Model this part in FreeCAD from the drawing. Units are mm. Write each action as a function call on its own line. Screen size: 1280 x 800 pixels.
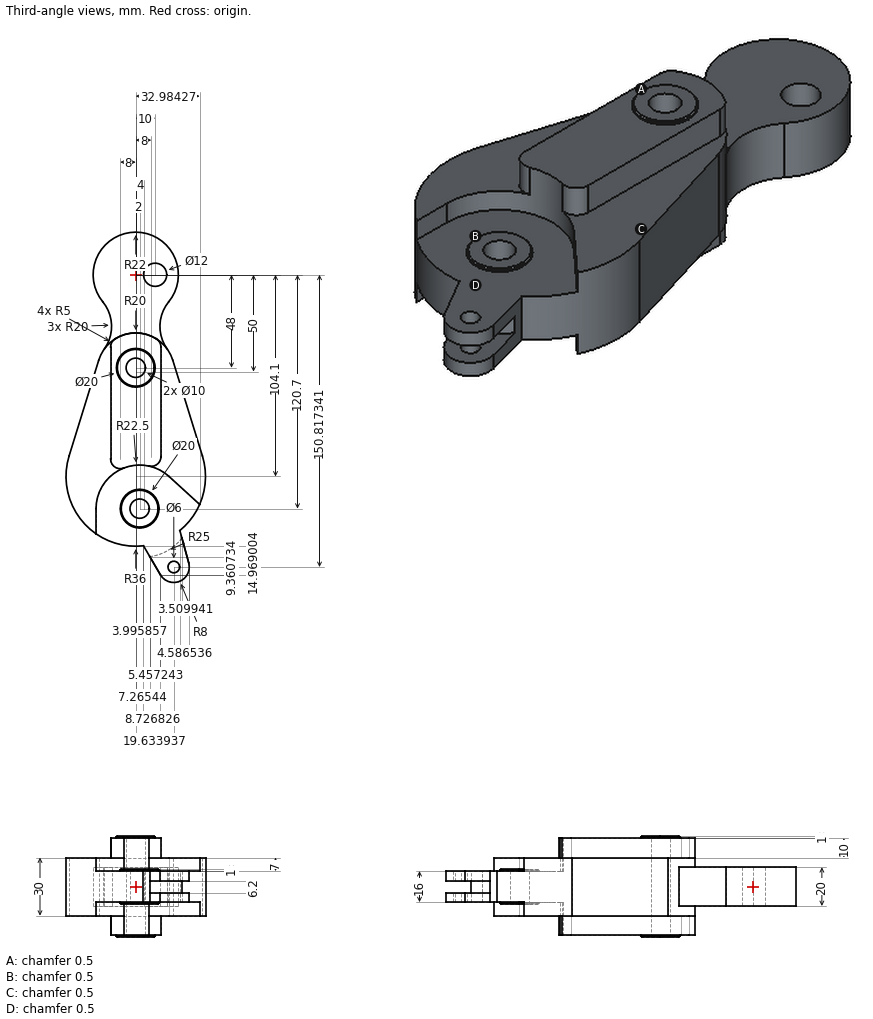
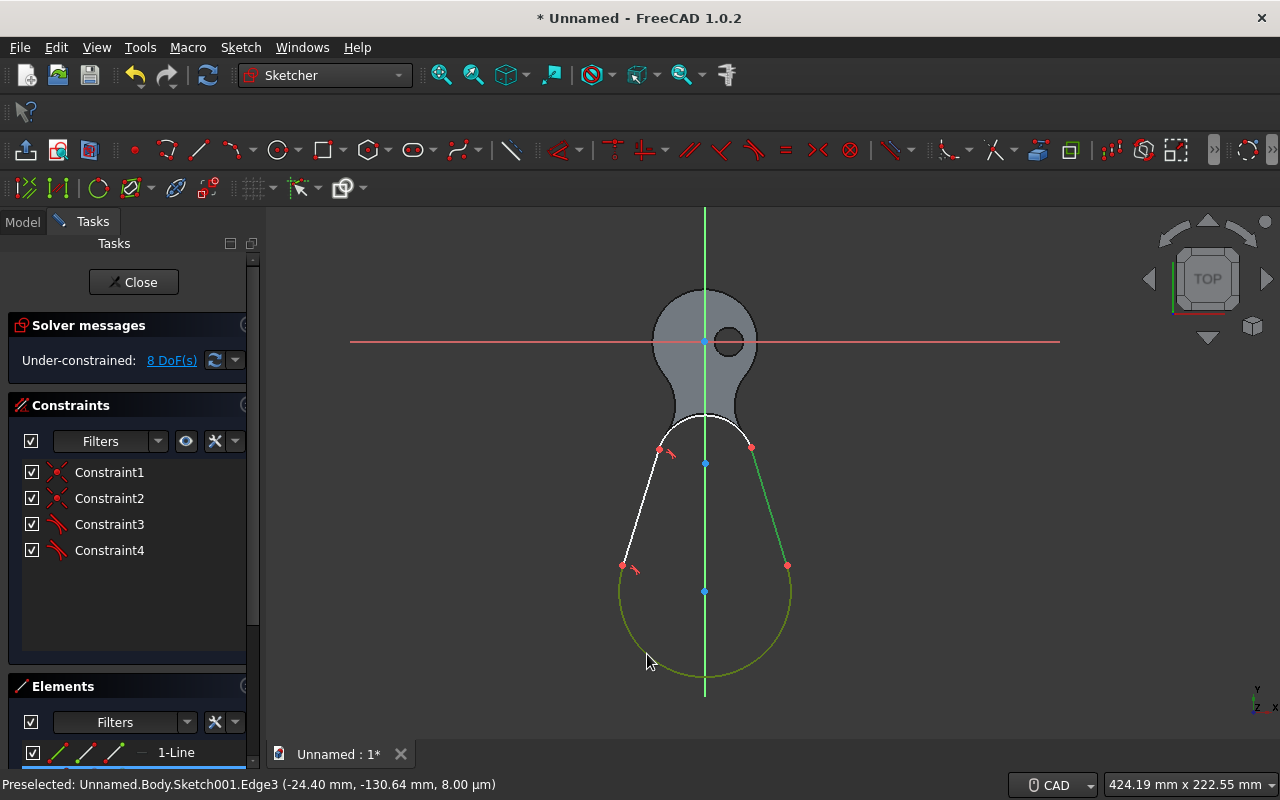
click(754, 150)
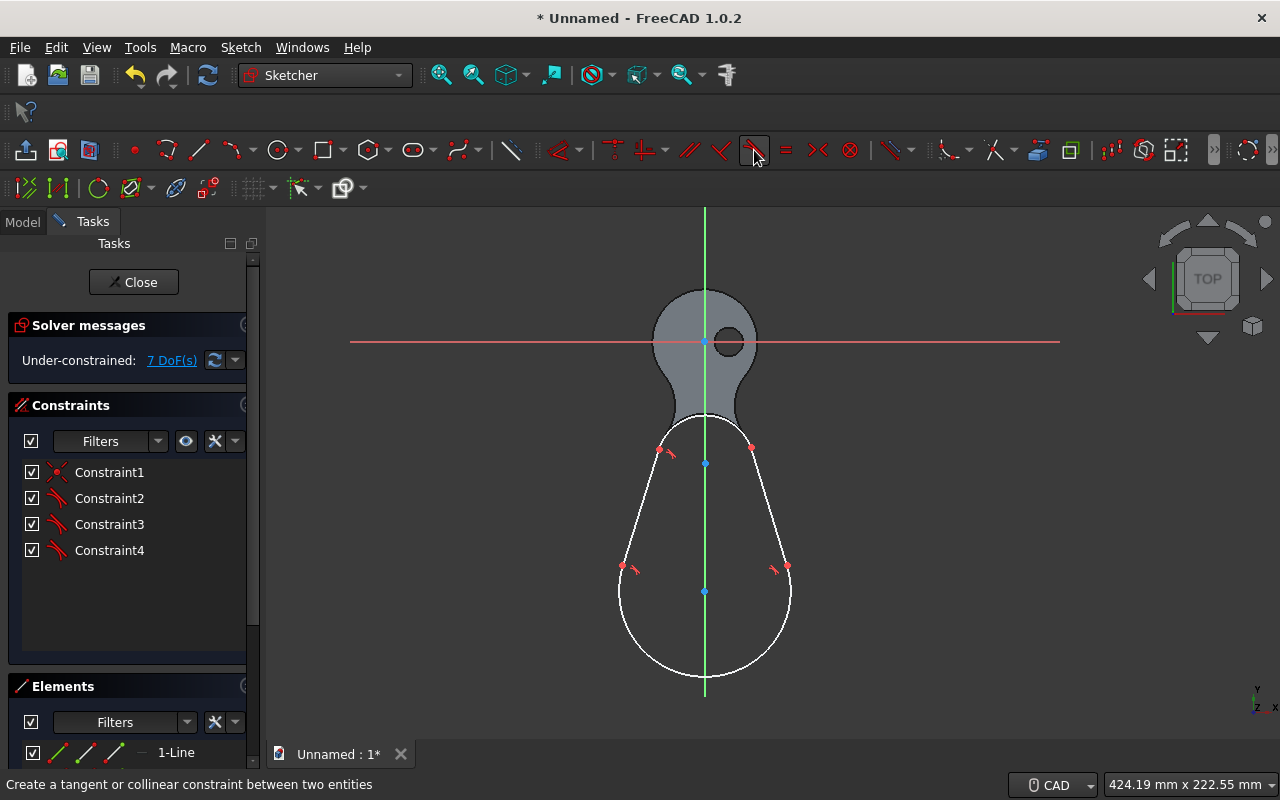
click(776, 531)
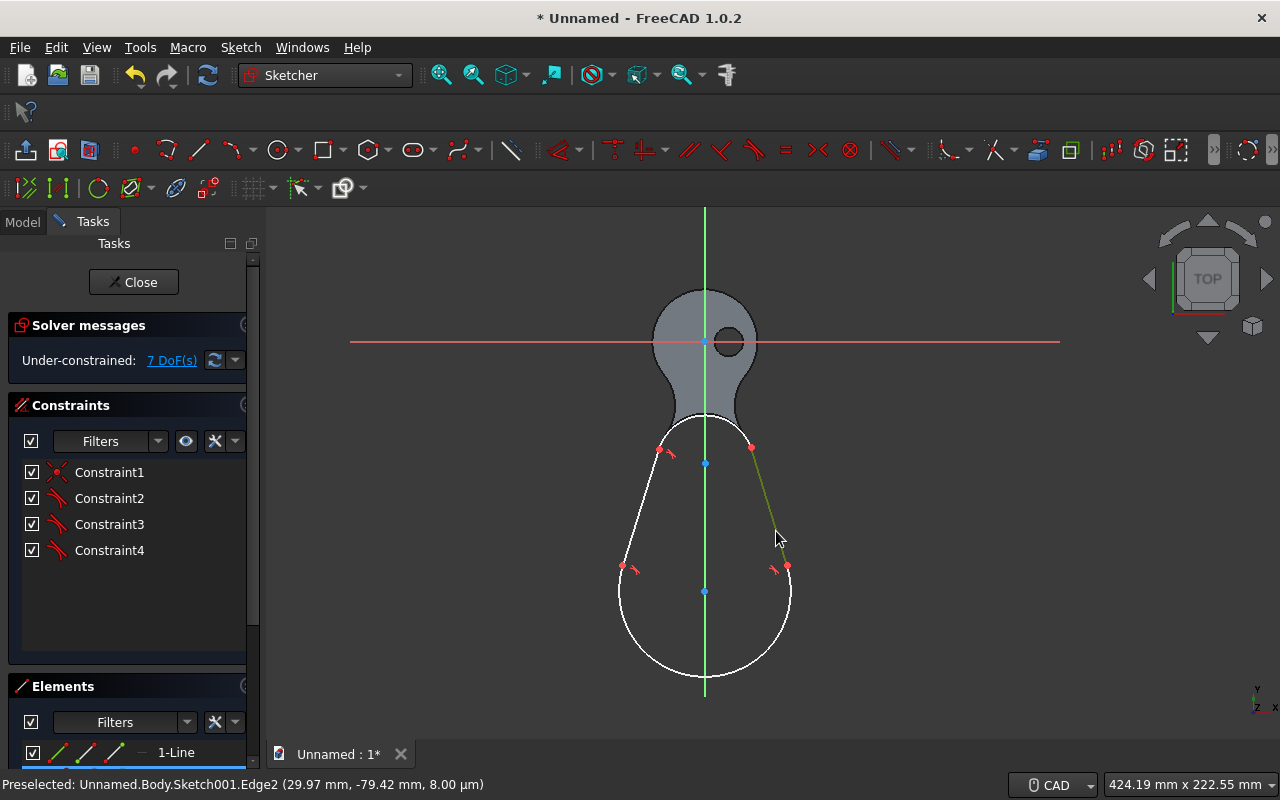
click(728, 421)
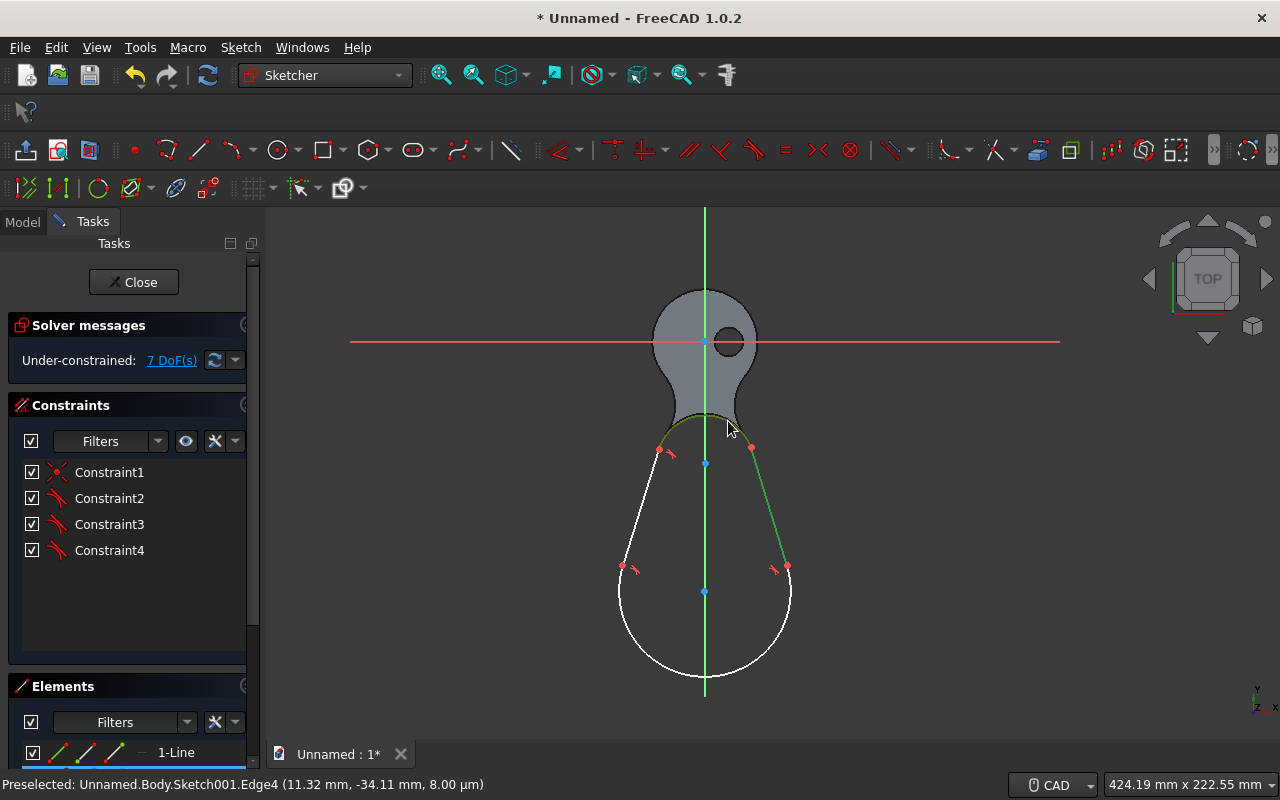
click(754, 150)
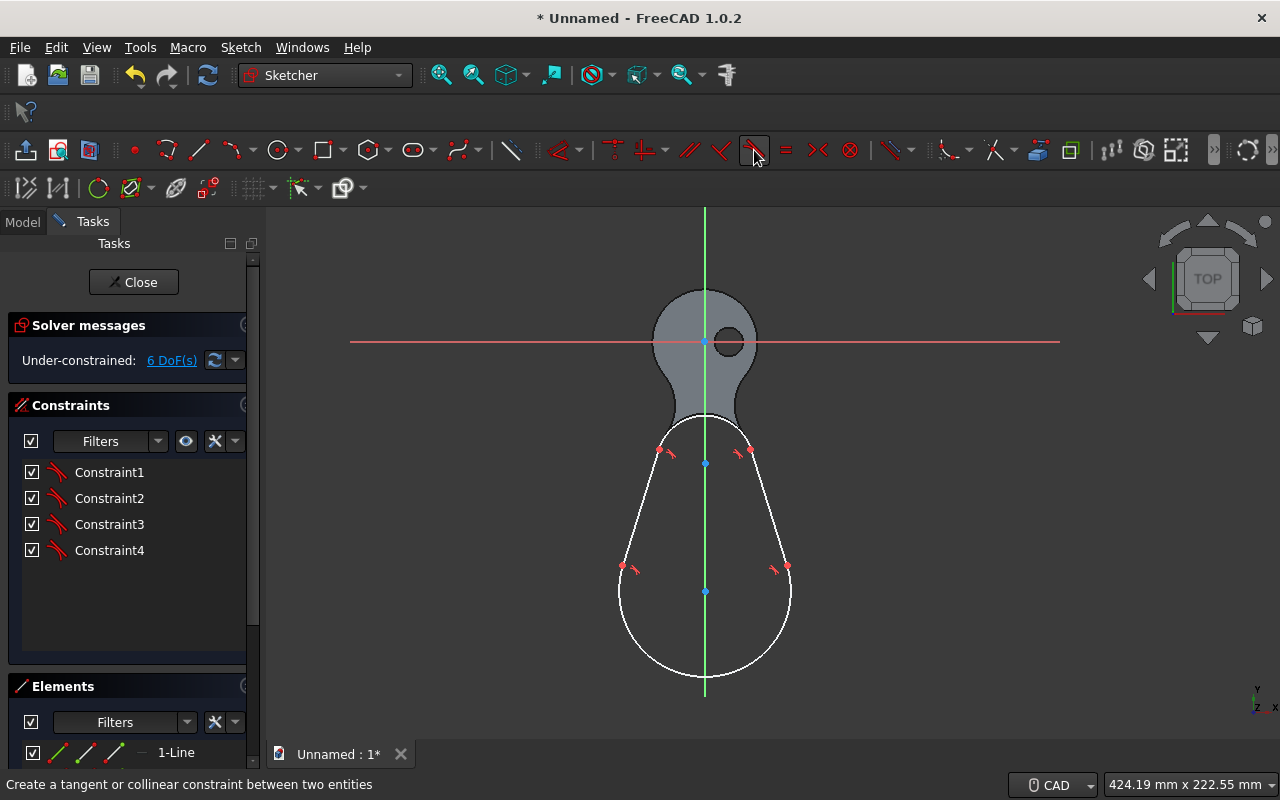
click(705, 591)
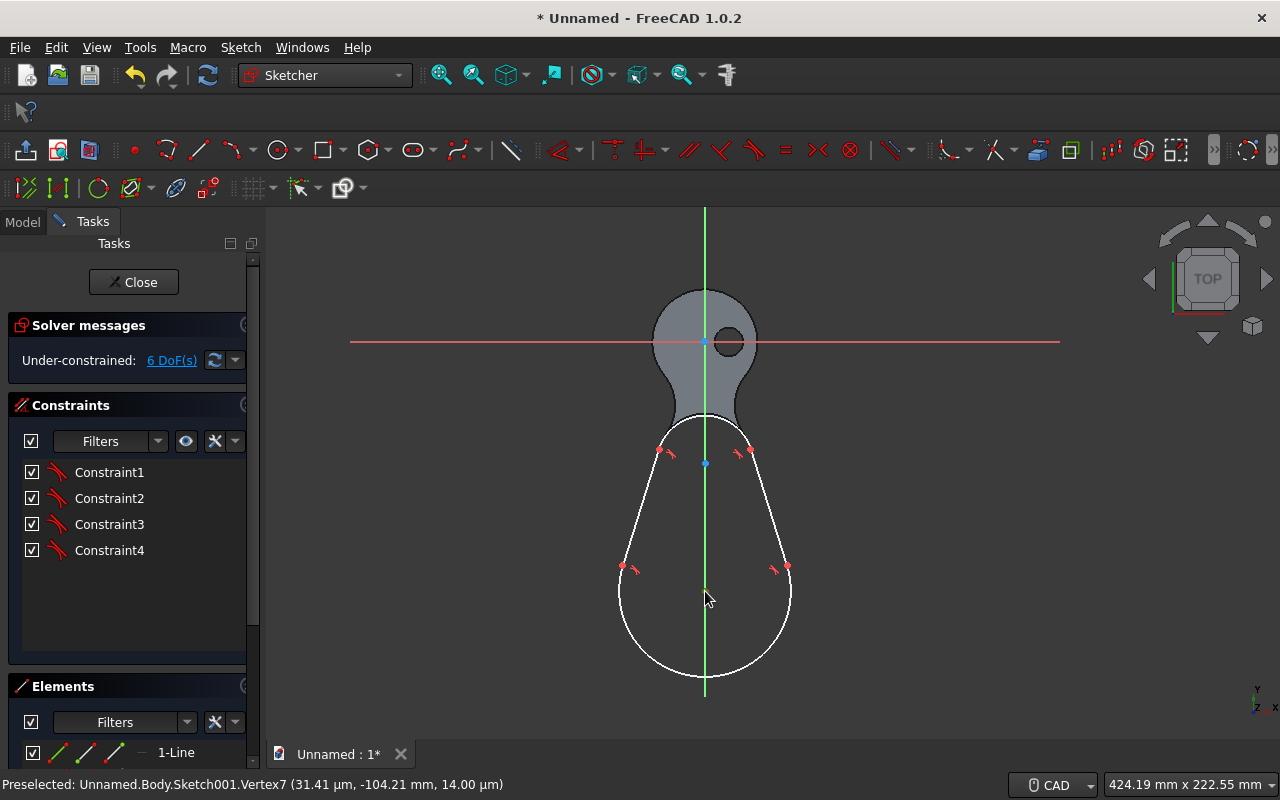
click(705, 643)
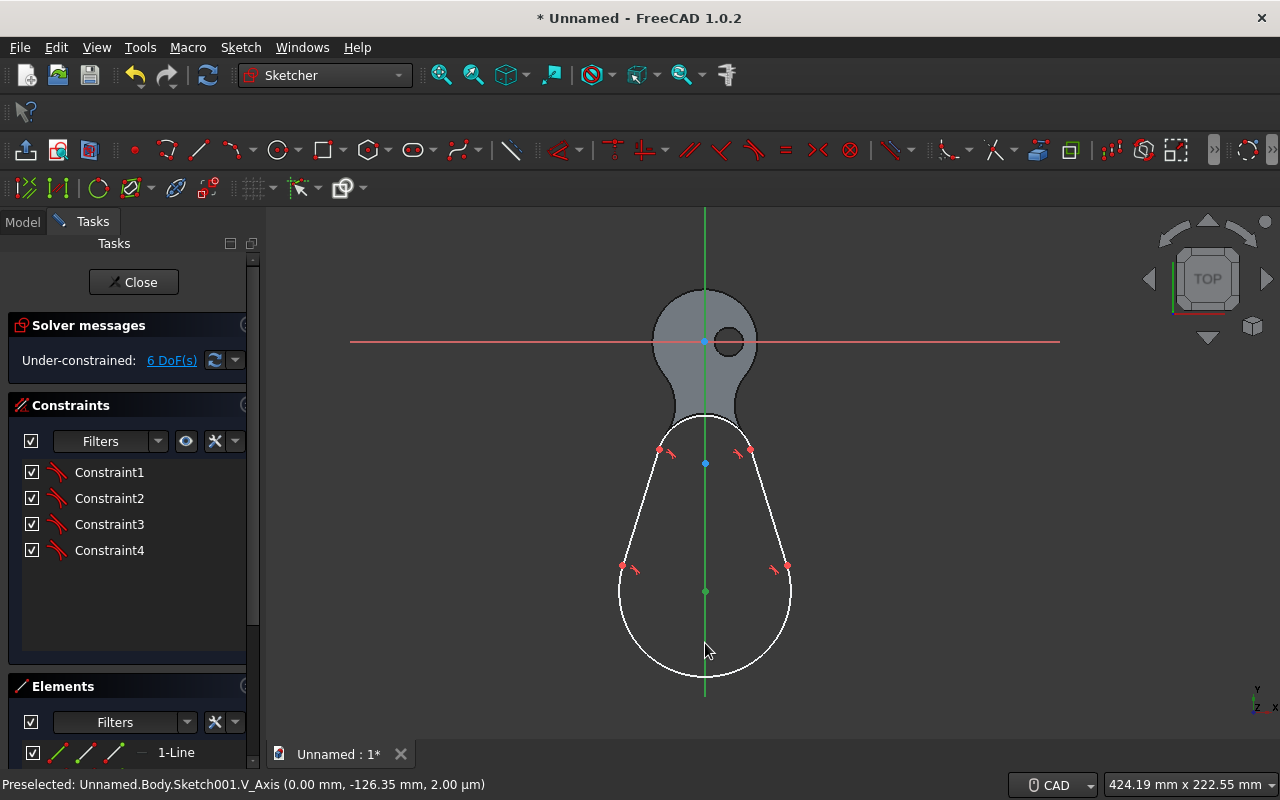
click(614, 150)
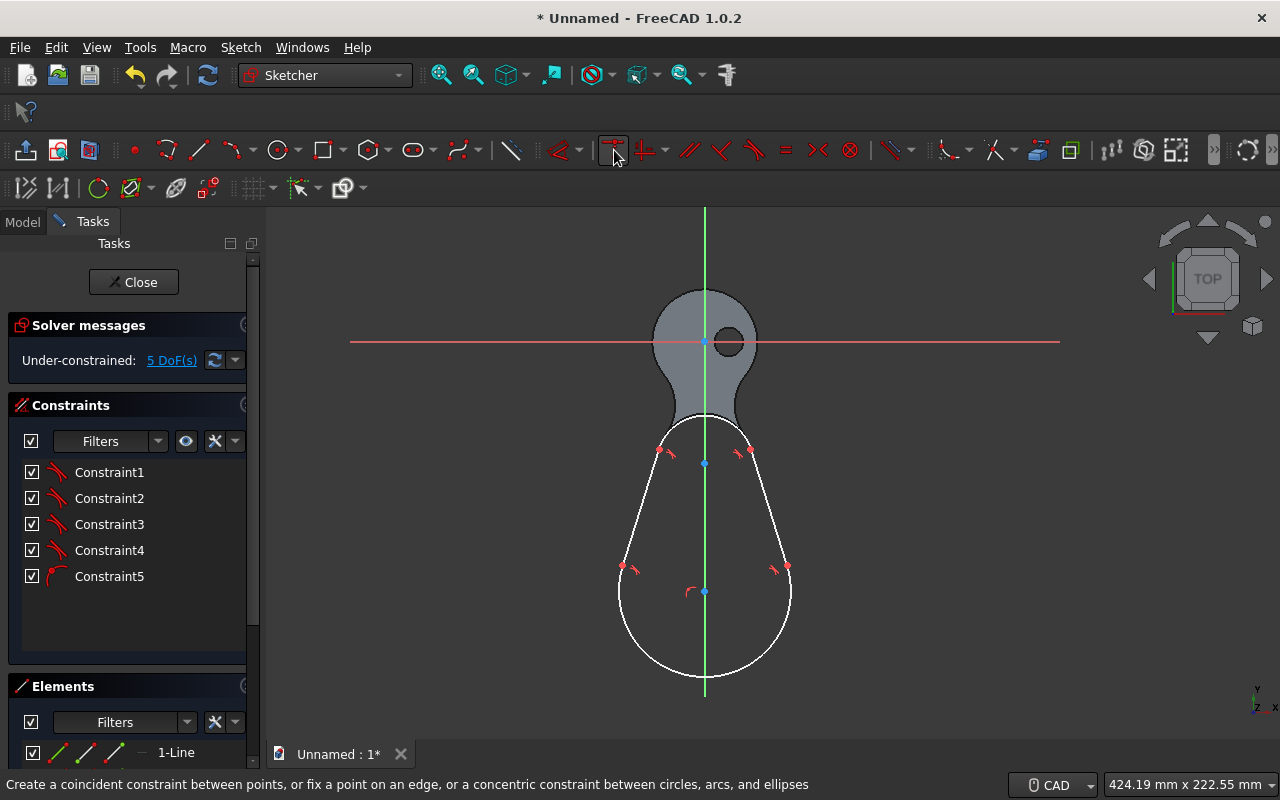
click(705, 464)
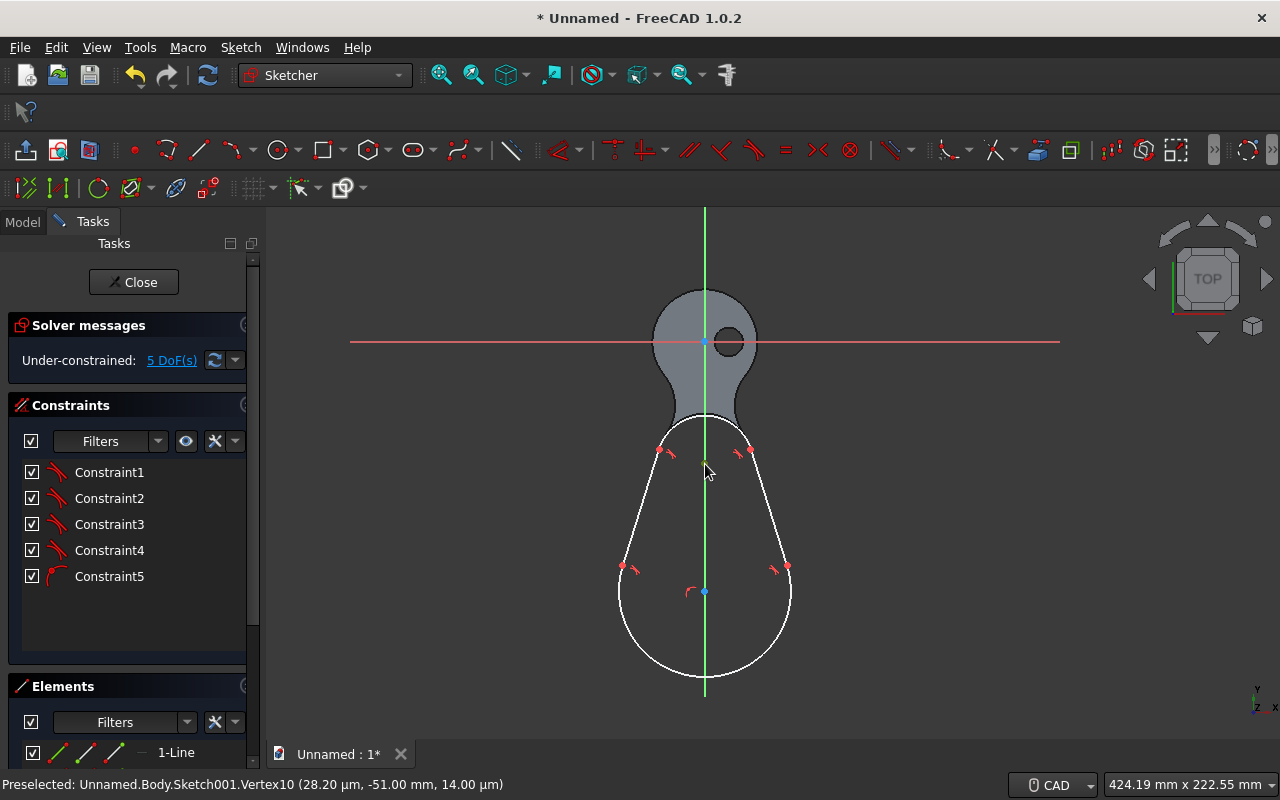
click(705, 643)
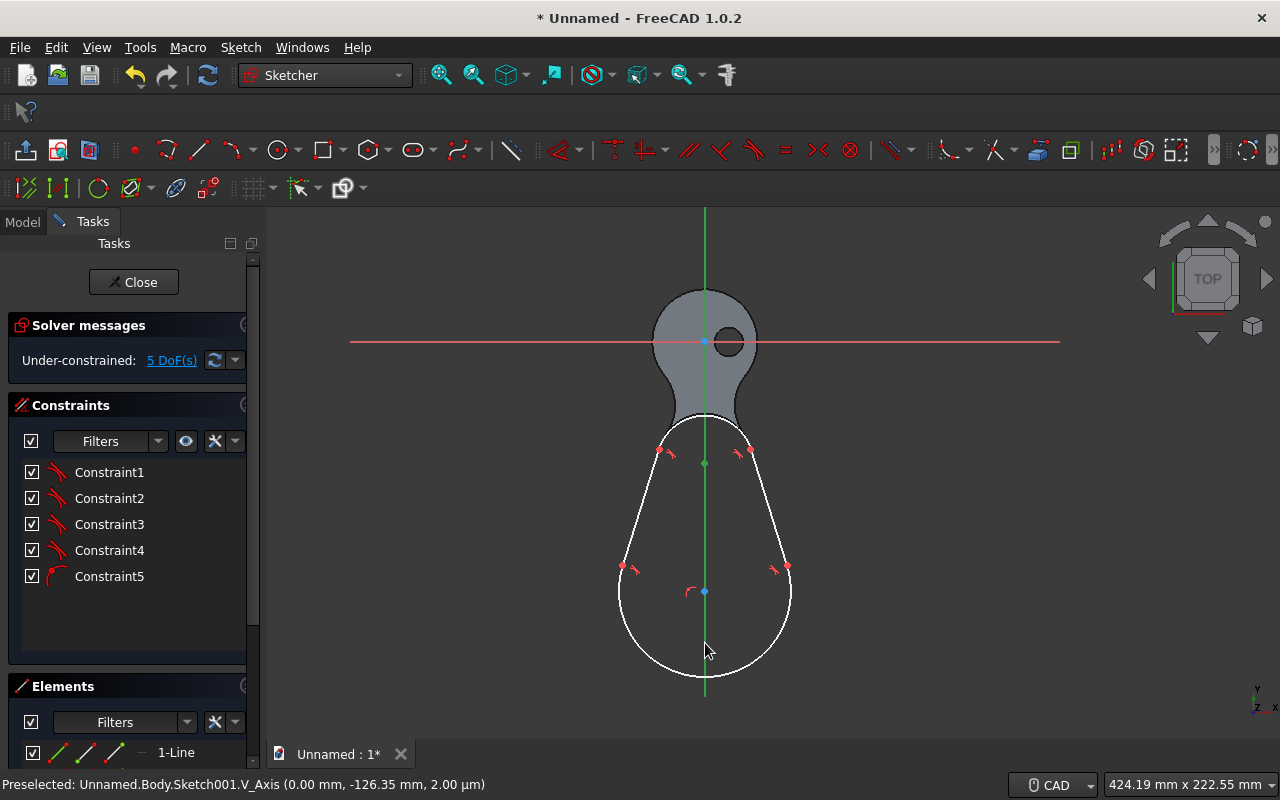
click(614, 150)